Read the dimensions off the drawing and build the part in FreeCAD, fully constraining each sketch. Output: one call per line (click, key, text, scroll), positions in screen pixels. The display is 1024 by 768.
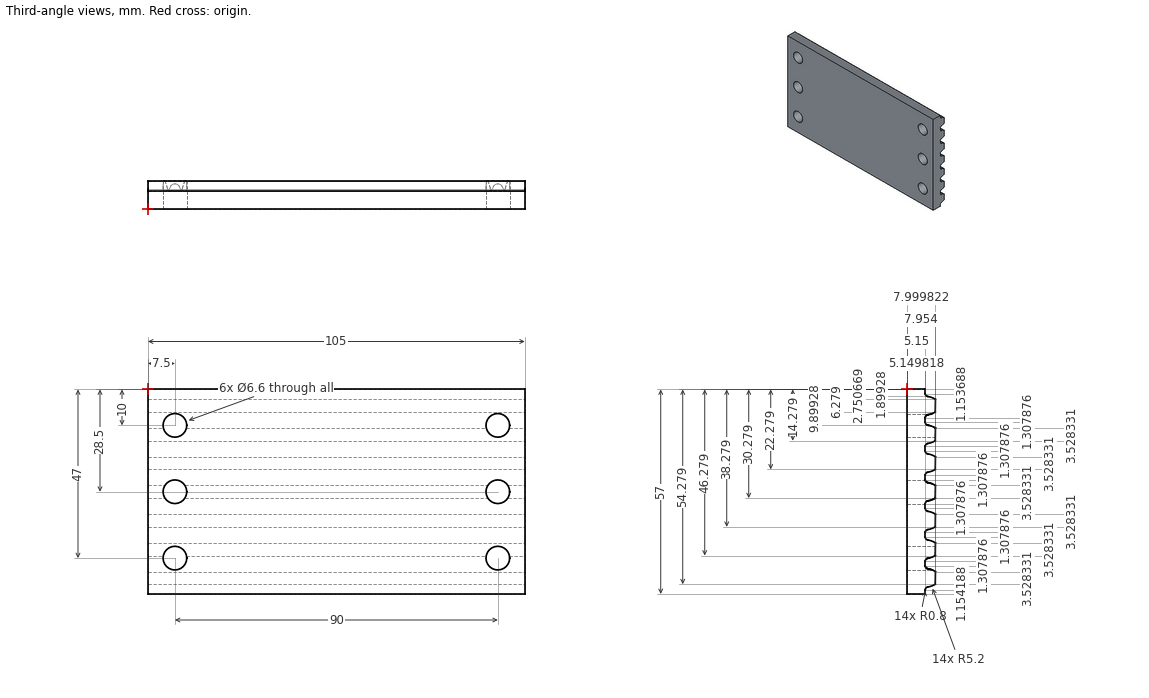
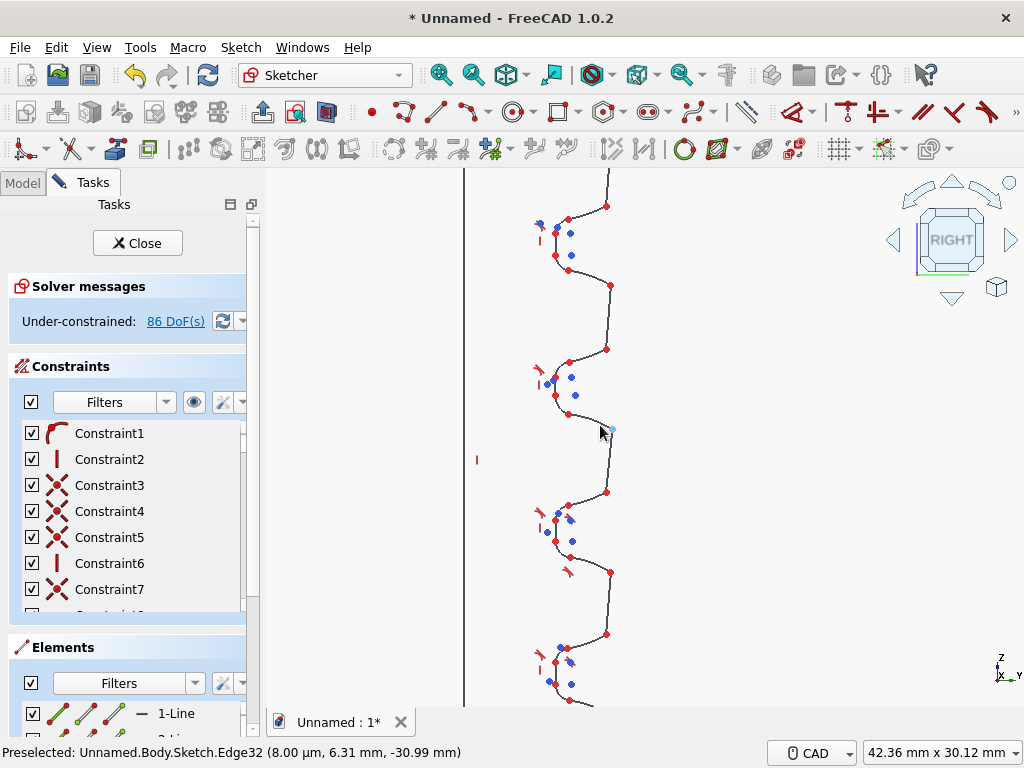
click(600, 423)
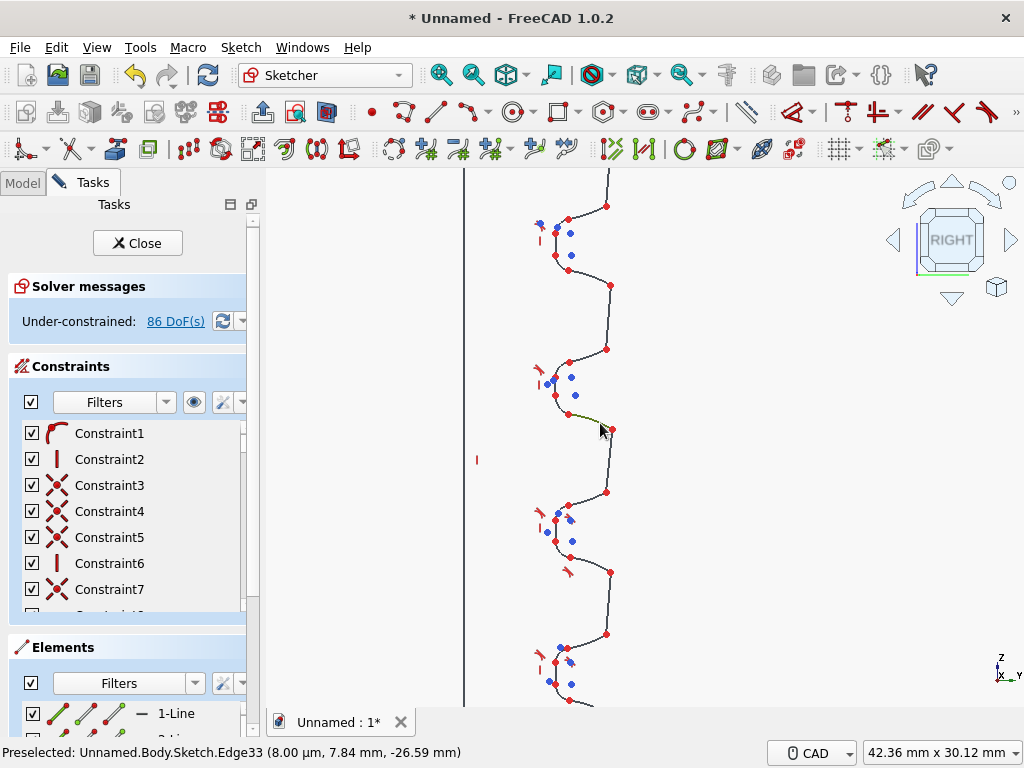
click(559, 407)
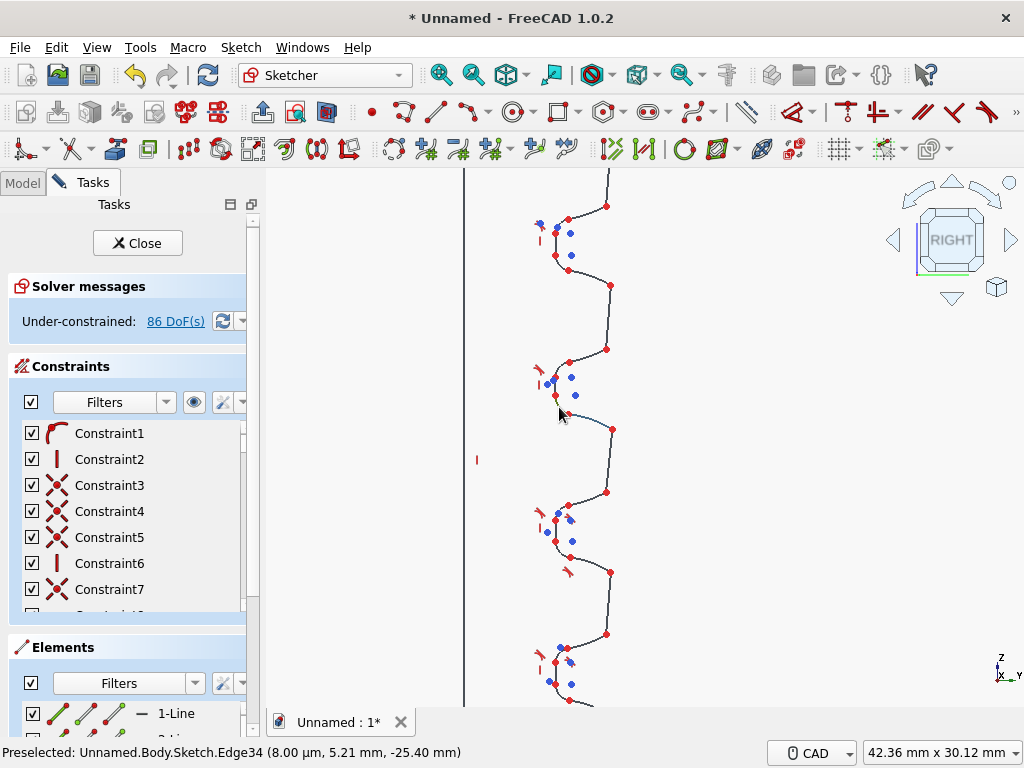
click(988, 112)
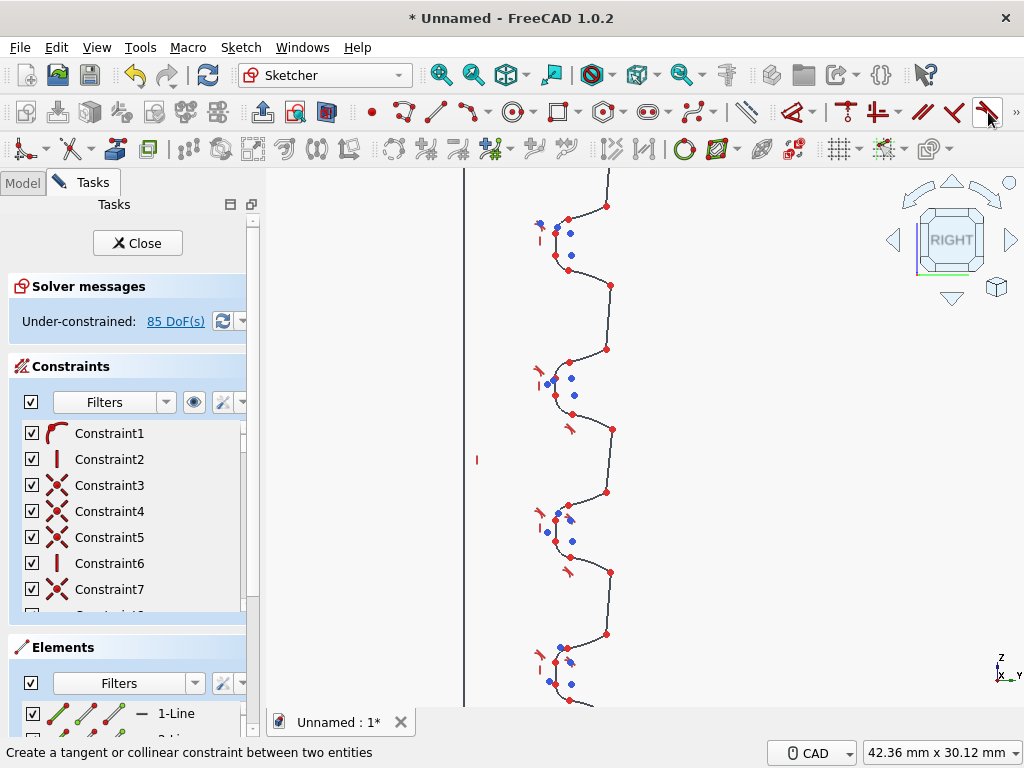
click(559, 367)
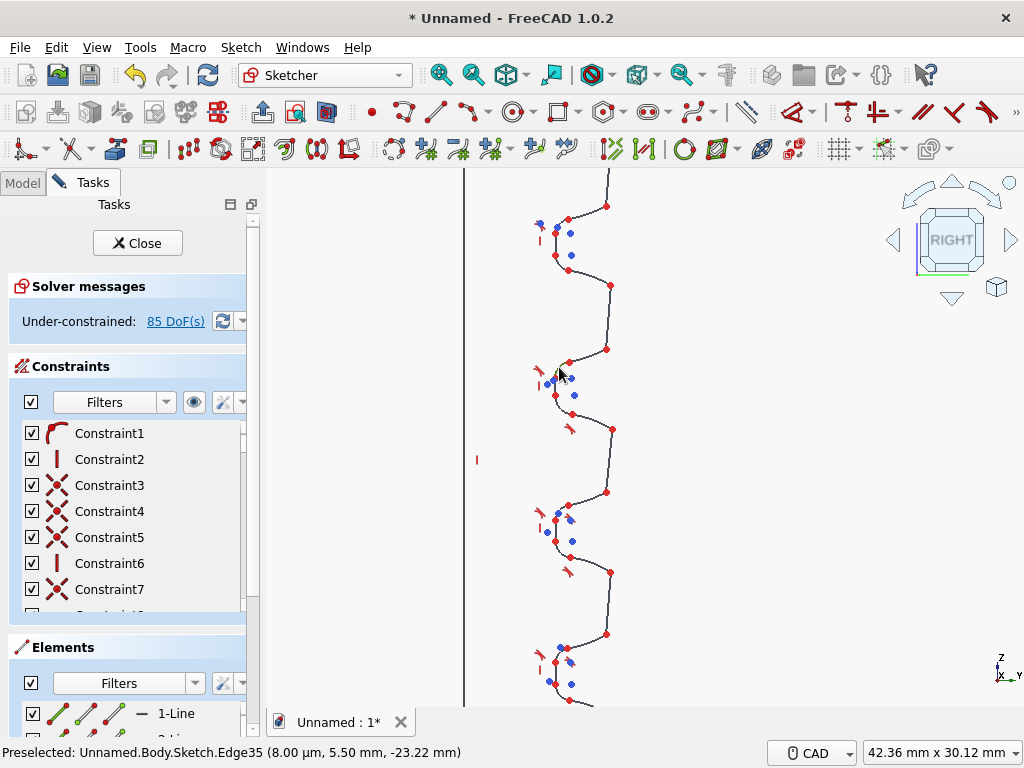
click(581, 359)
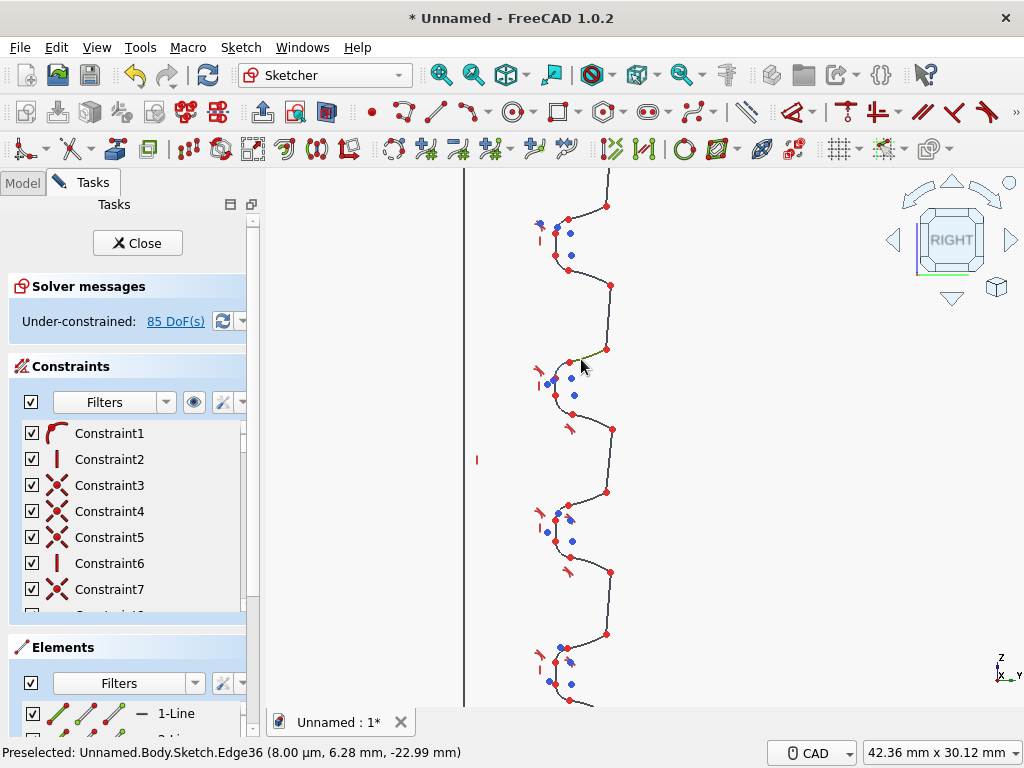
click(988, 112)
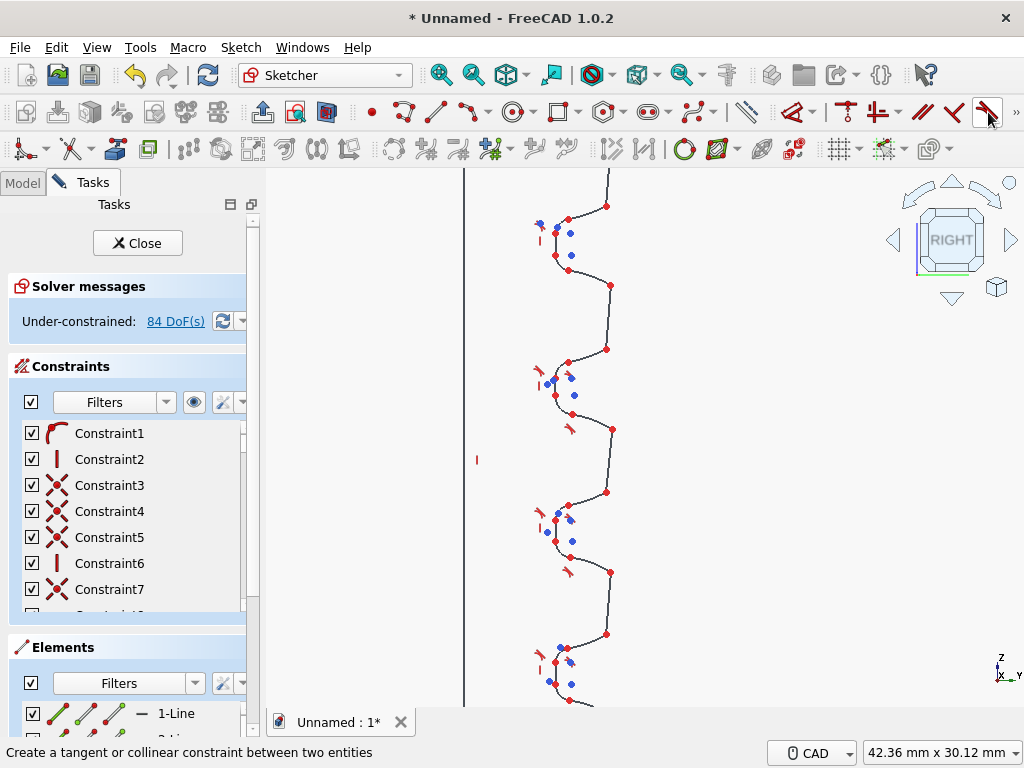
click(599, 279)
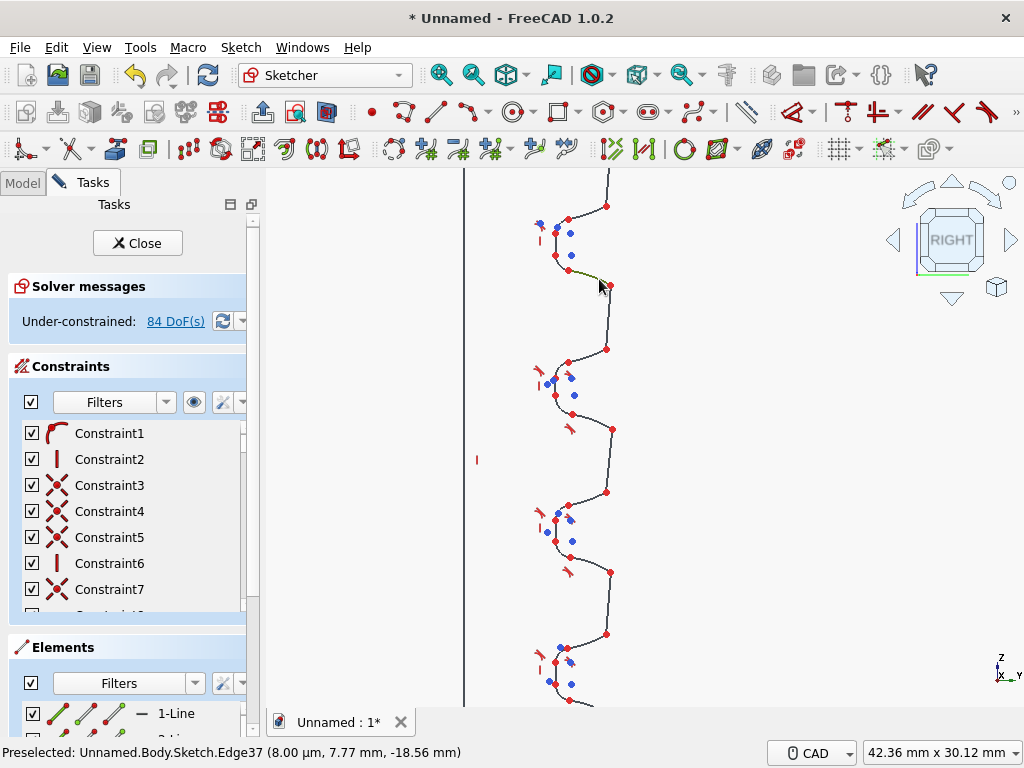
scroll(560, 265, up, 2)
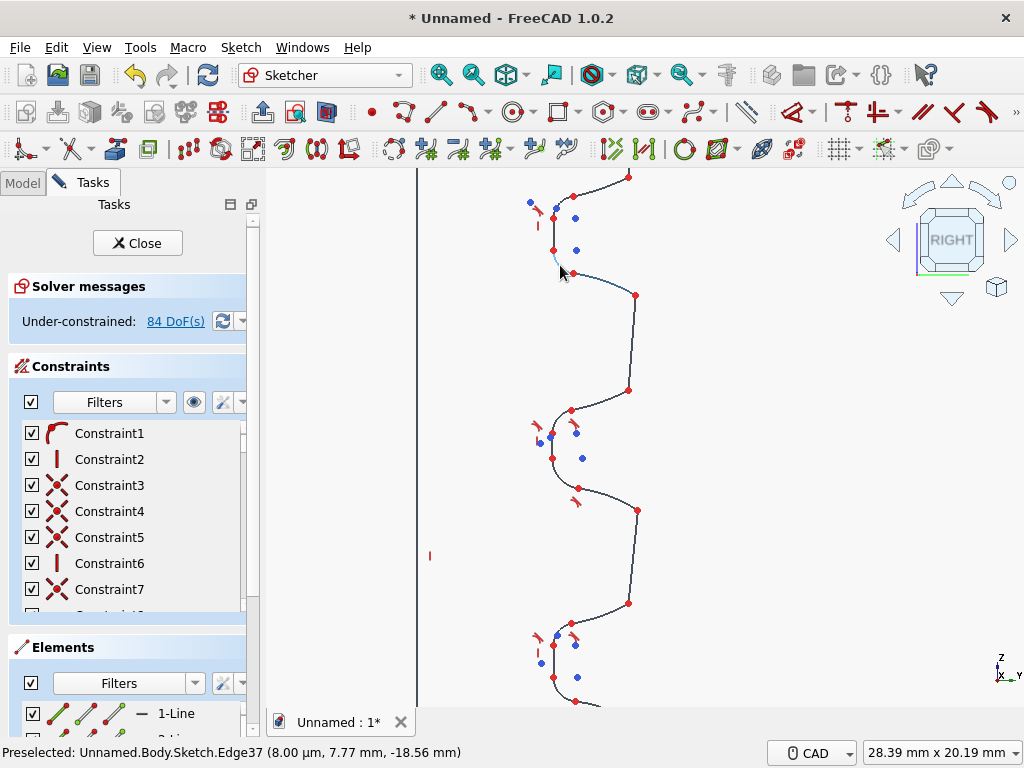
click(559, 266)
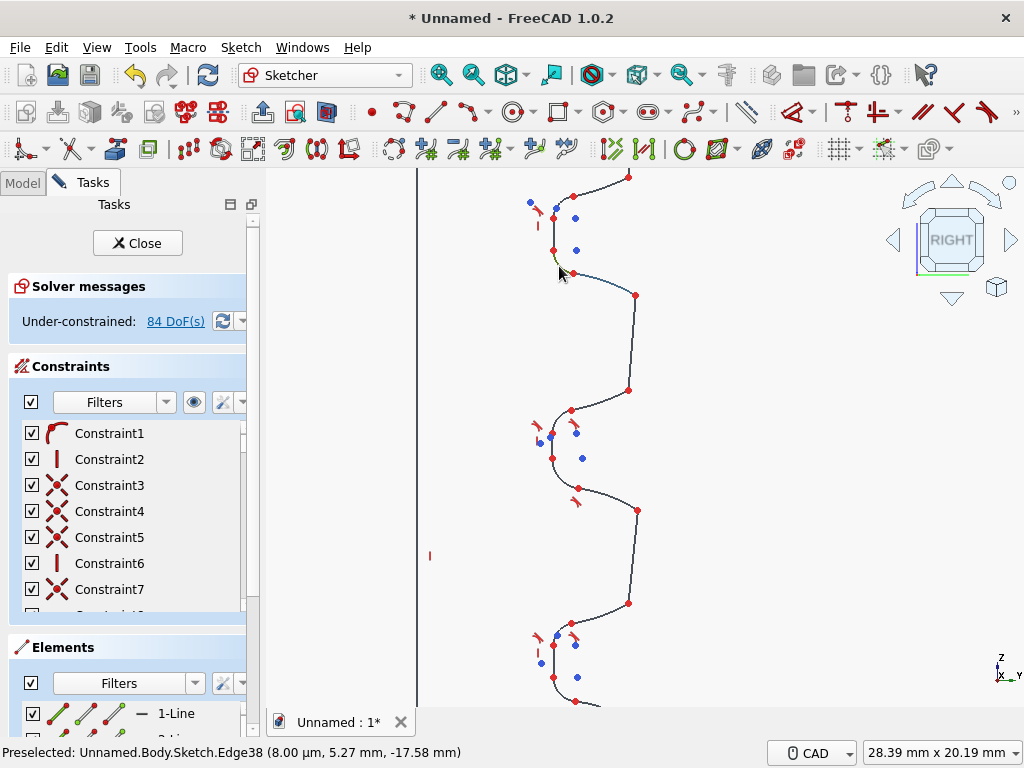
click(988, 112)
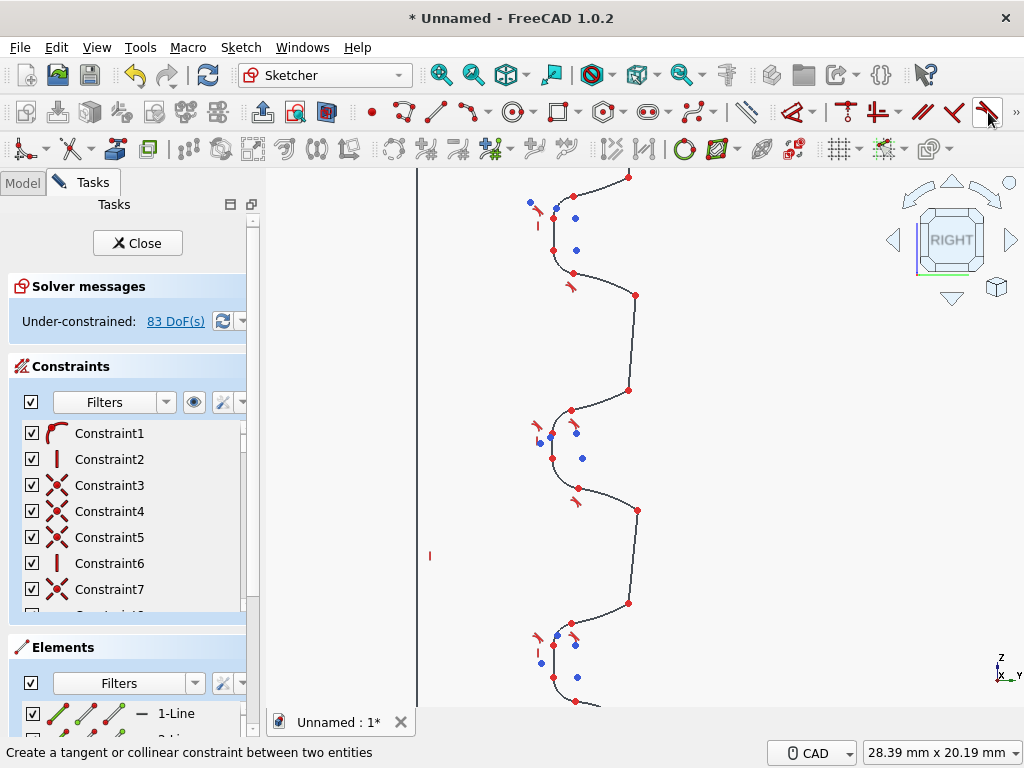
scroll(564, 200, up, 2)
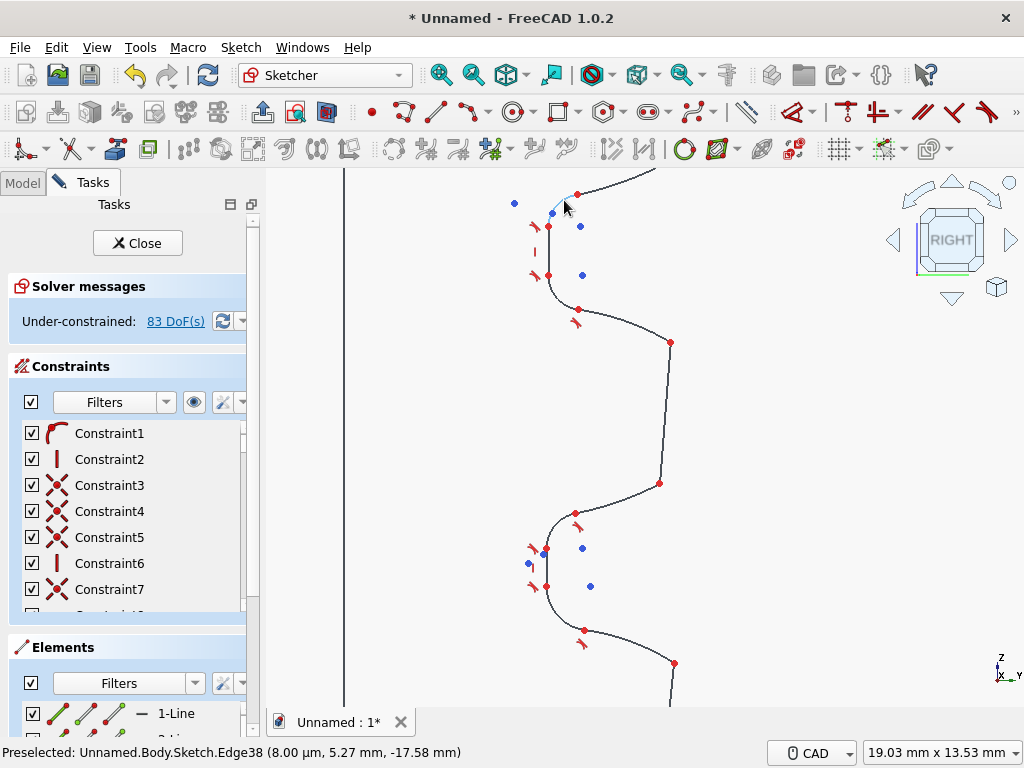
click(564, 199)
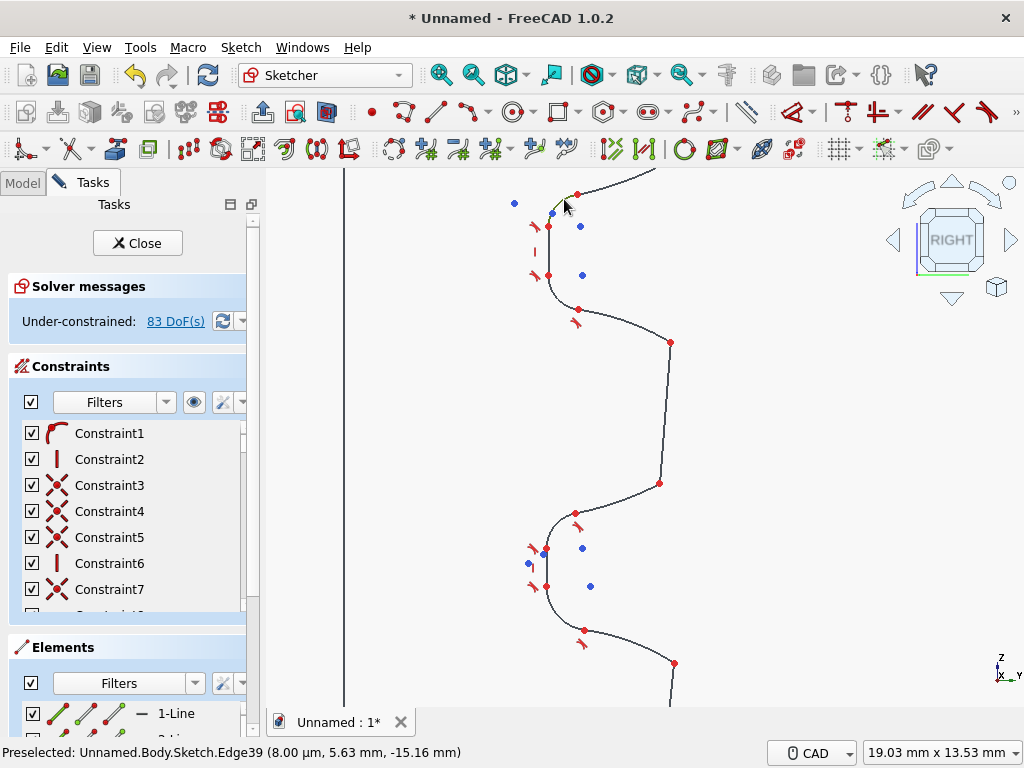
scroll(591, 380, down, 9)